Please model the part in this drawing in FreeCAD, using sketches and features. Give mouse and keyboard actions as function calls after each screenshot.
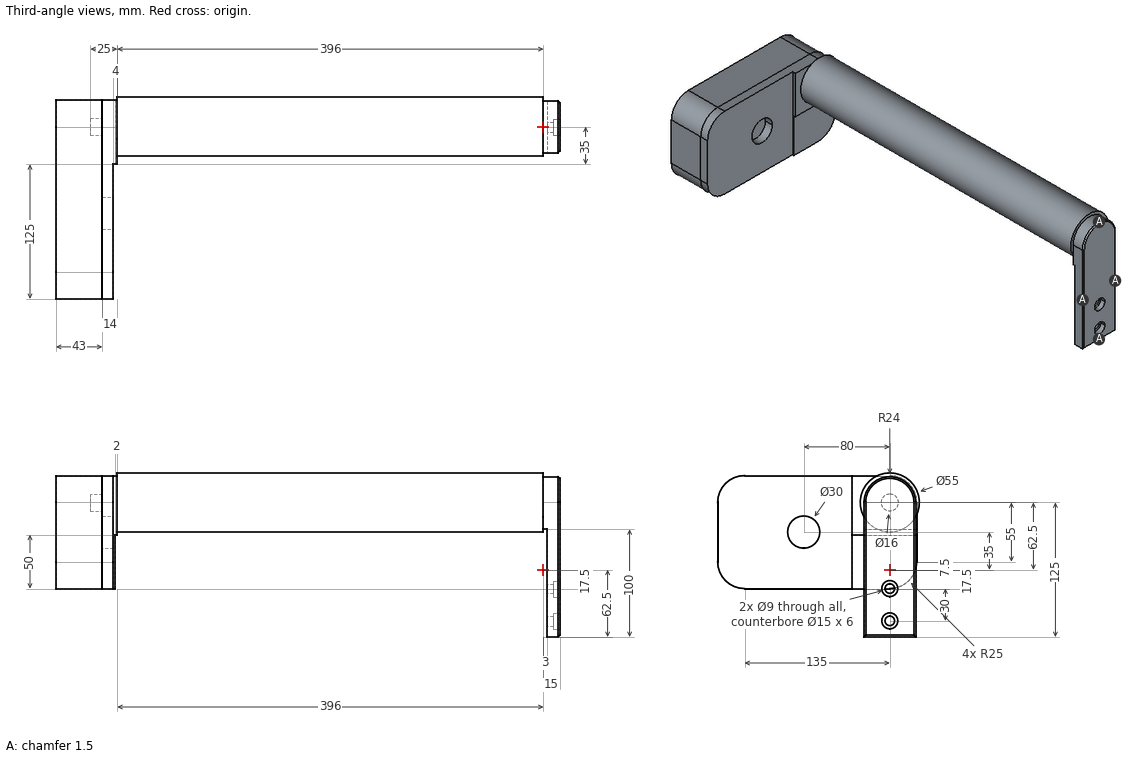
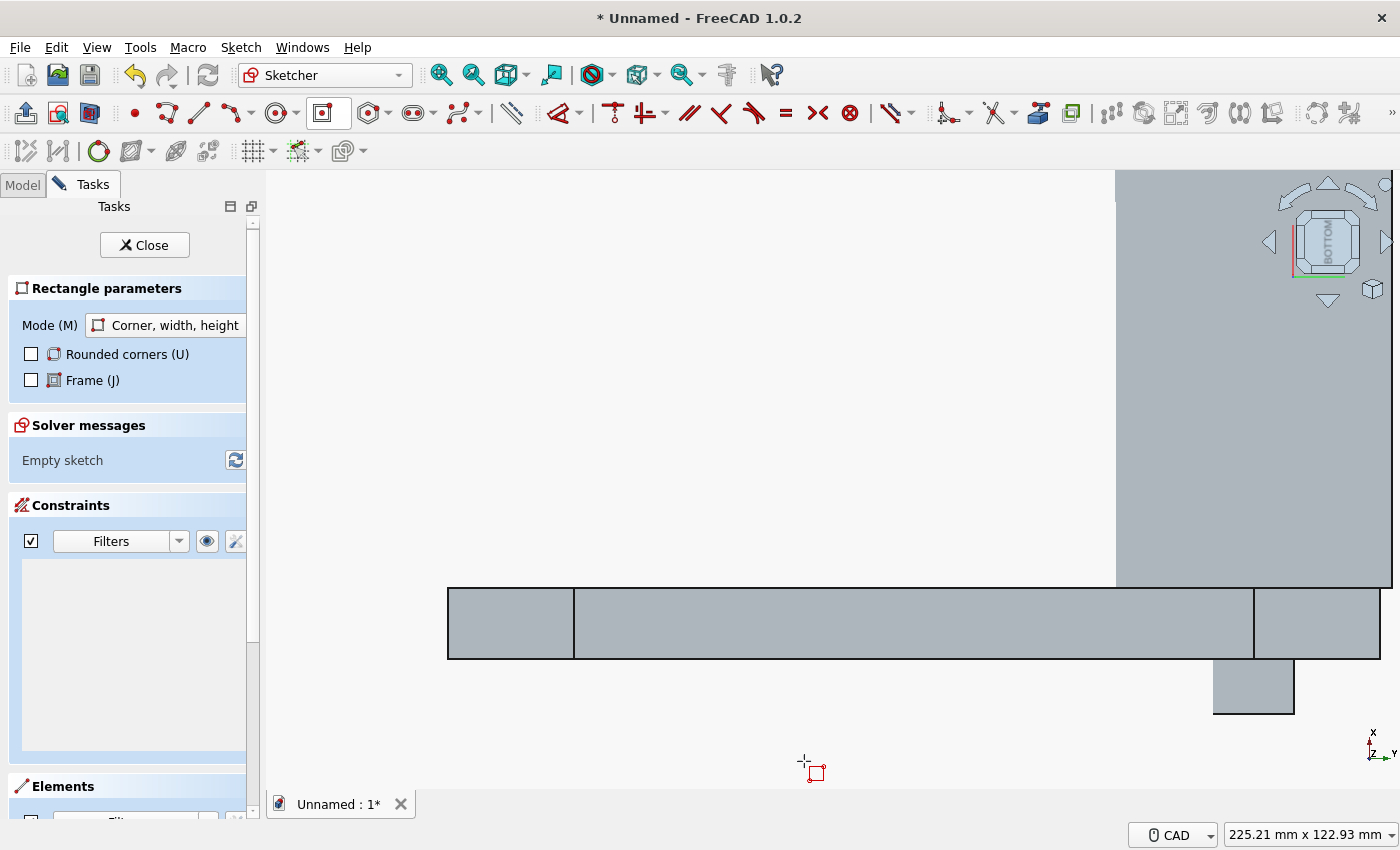
click(448, 588)
move(1078, 609)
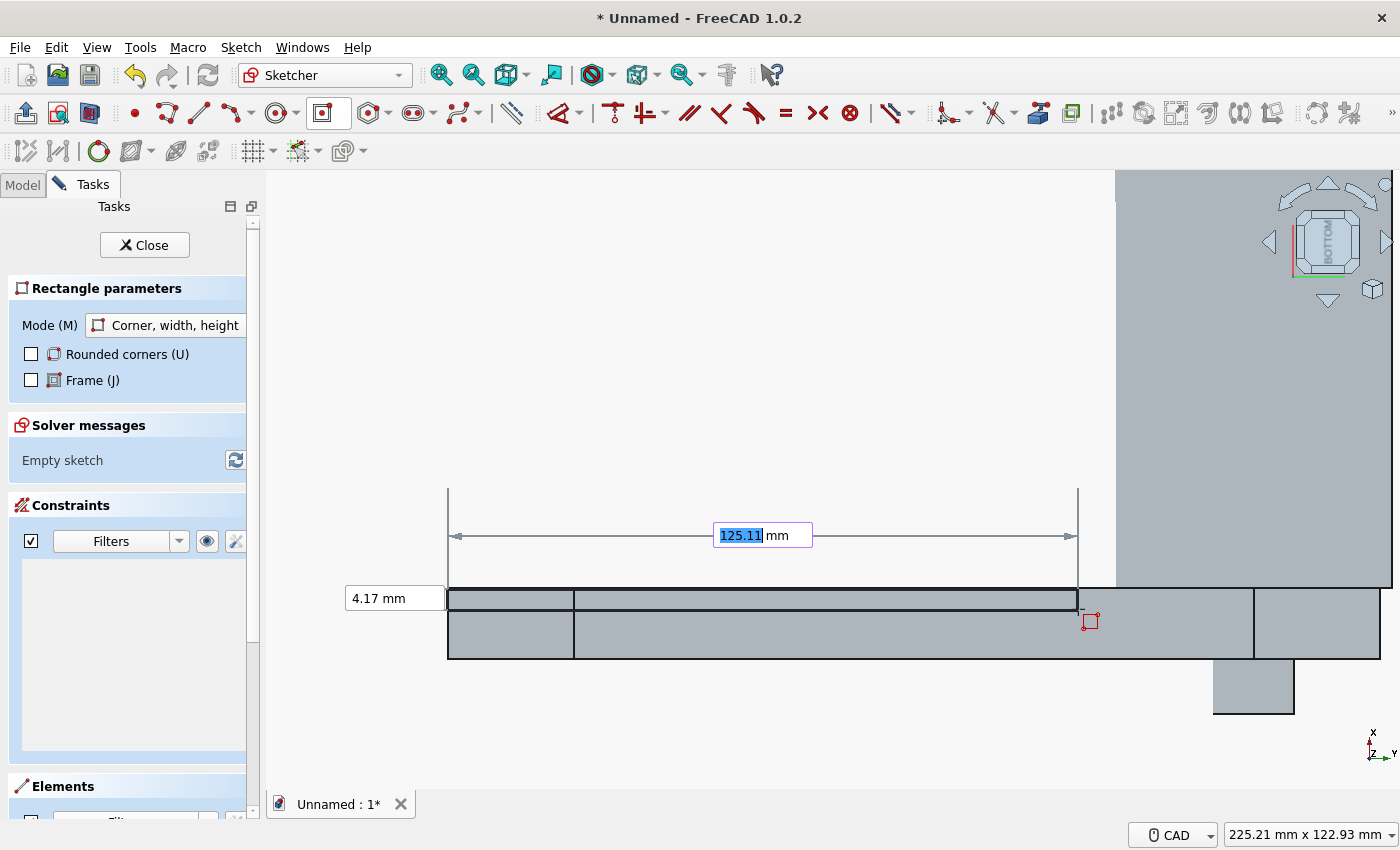
text(125)
key(Tab)
text(4)
key(Return)
key(Escape)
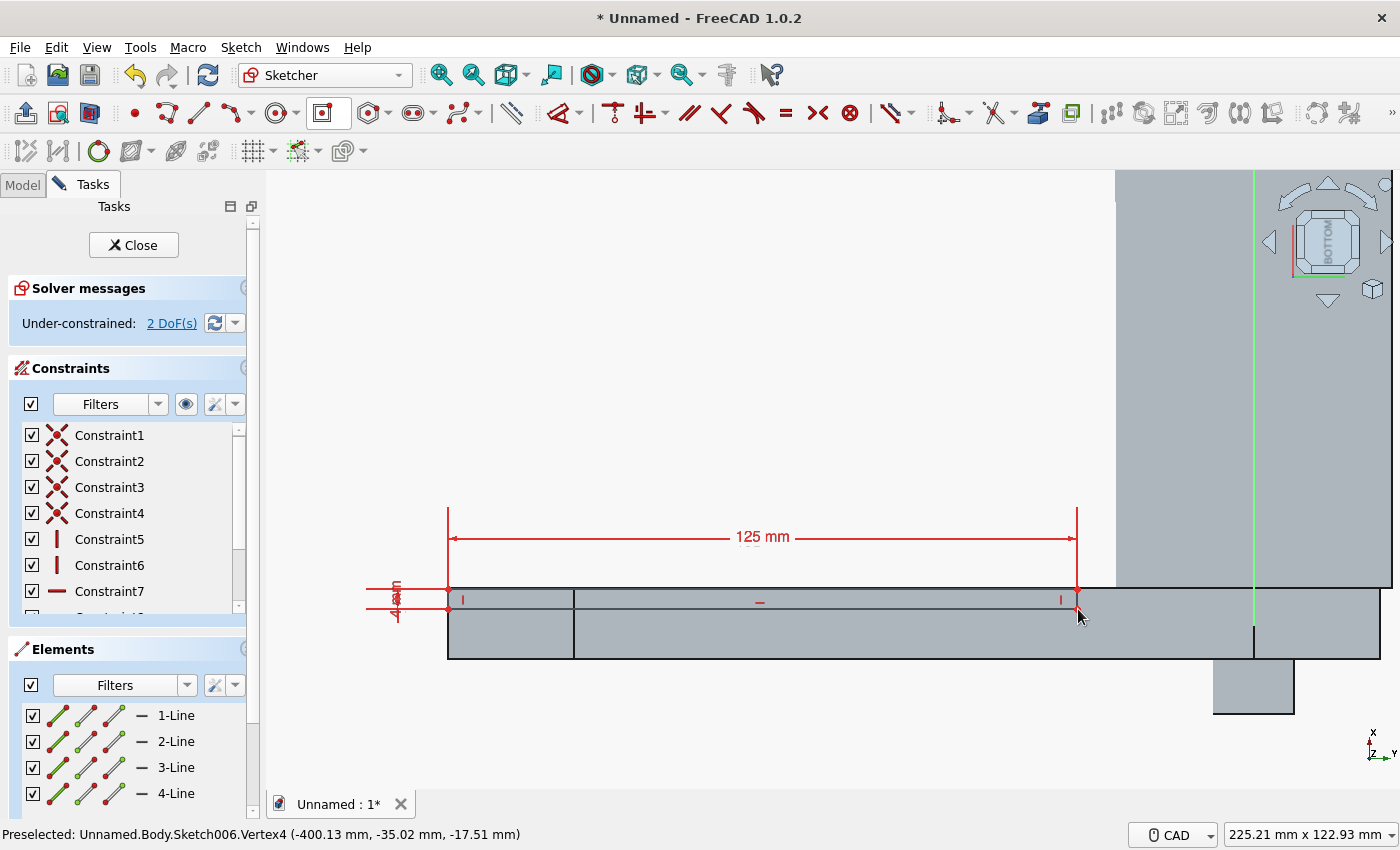
click(558, 114)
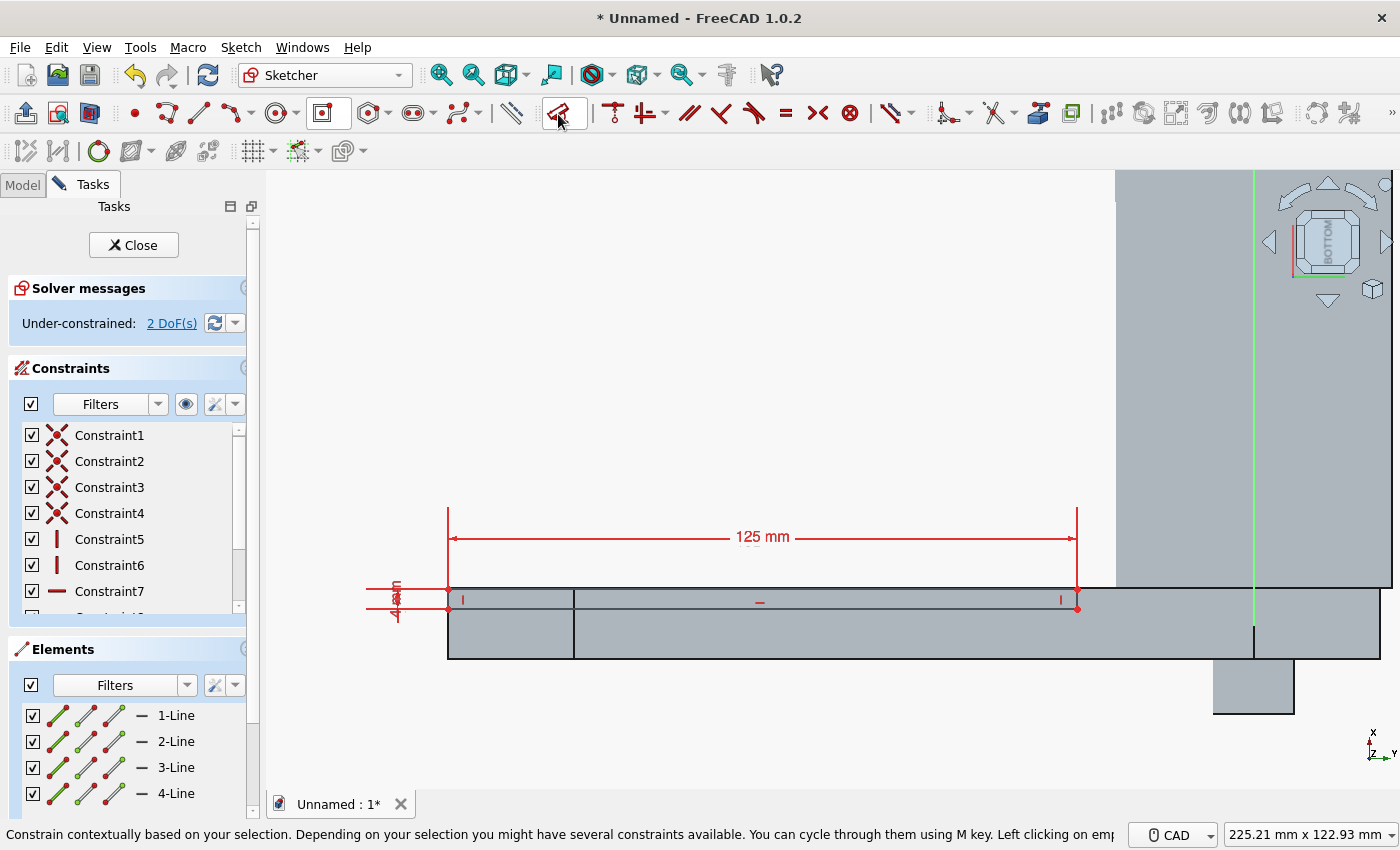
click(1077, 609)
click(1156, 643)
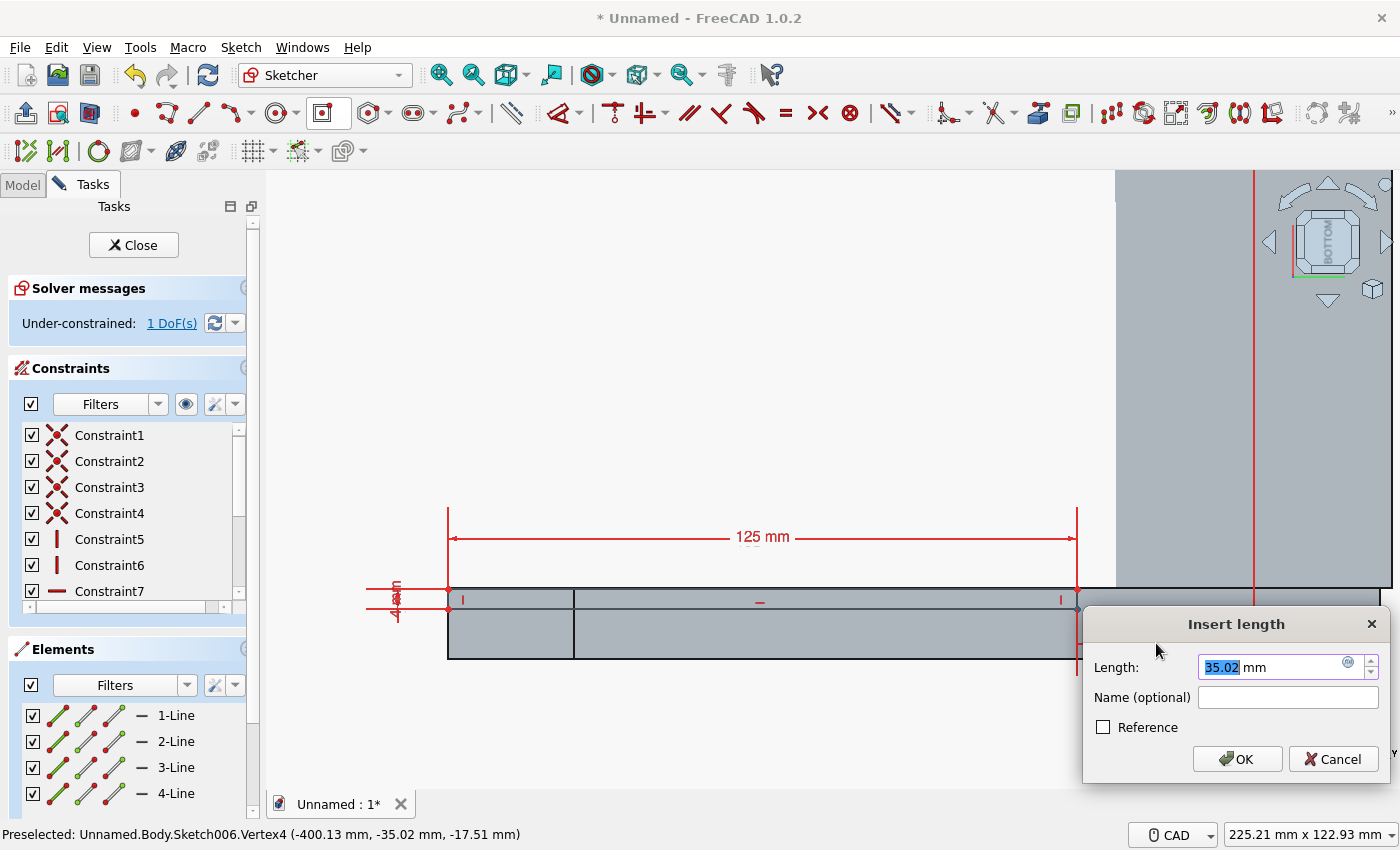
text(35)
key(Return)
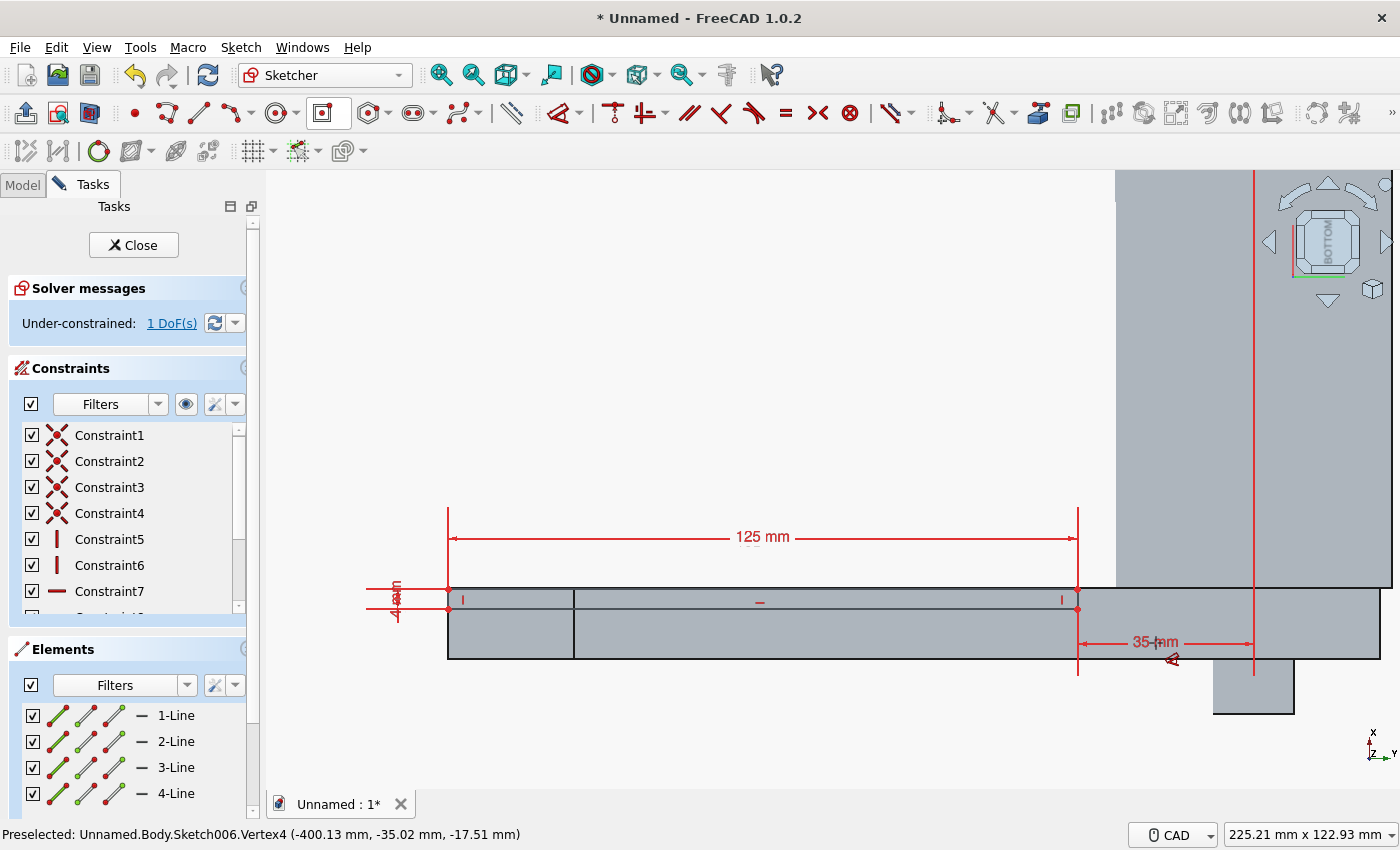
click(448, 589)
click(414, 394)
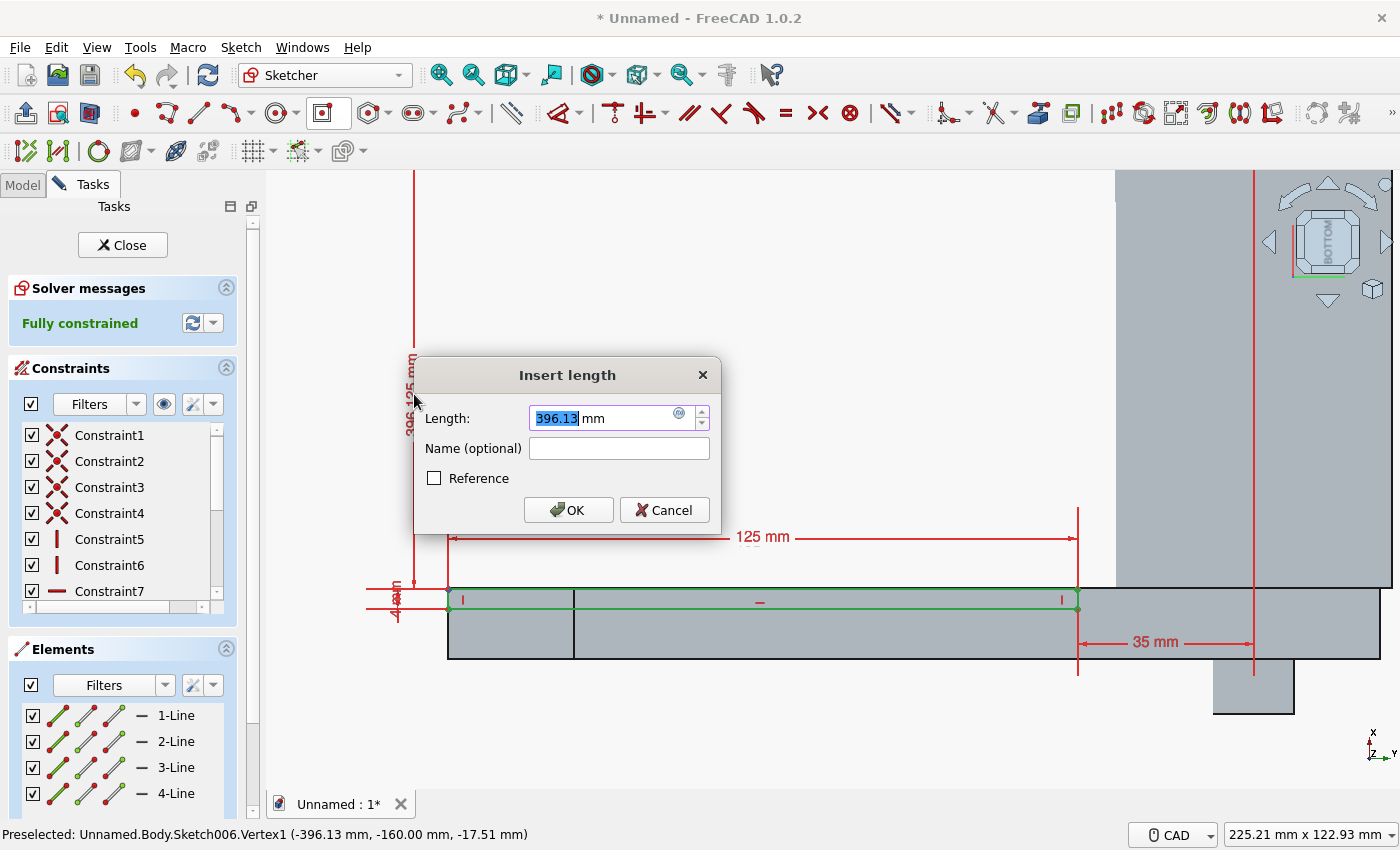
text(396)
key(Return)
key(Escape)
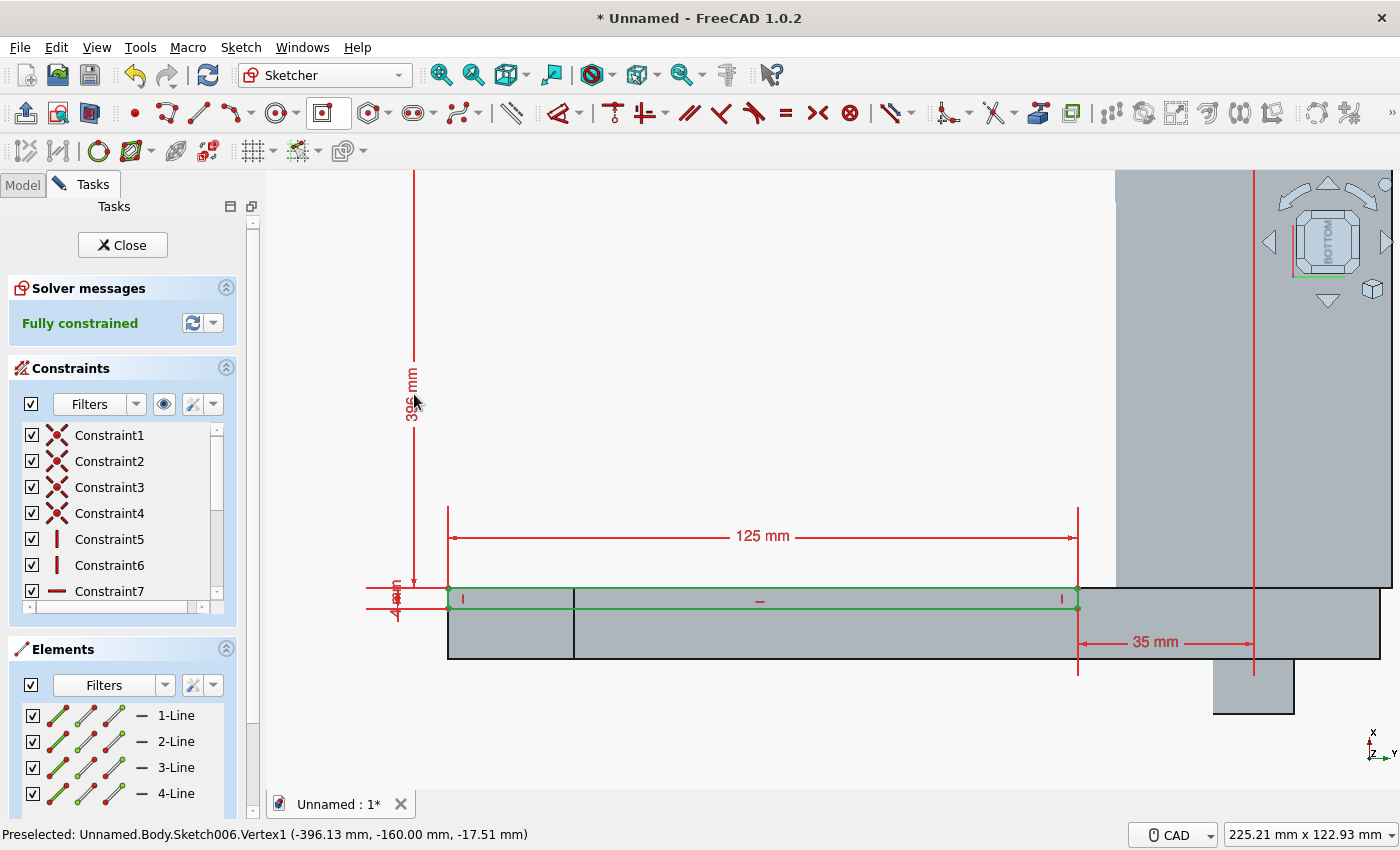
click(123, 245)